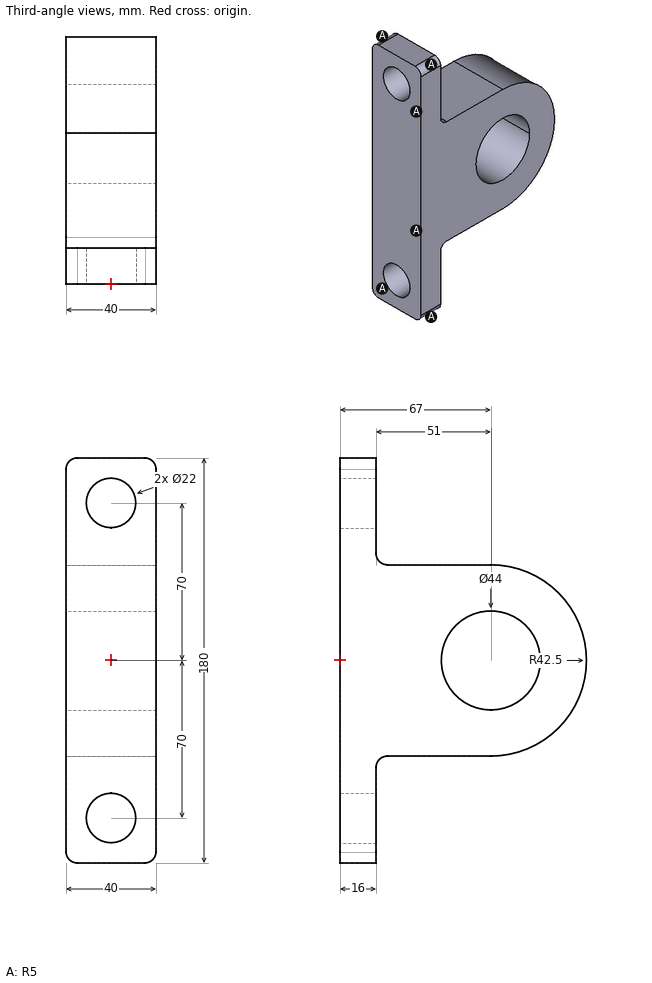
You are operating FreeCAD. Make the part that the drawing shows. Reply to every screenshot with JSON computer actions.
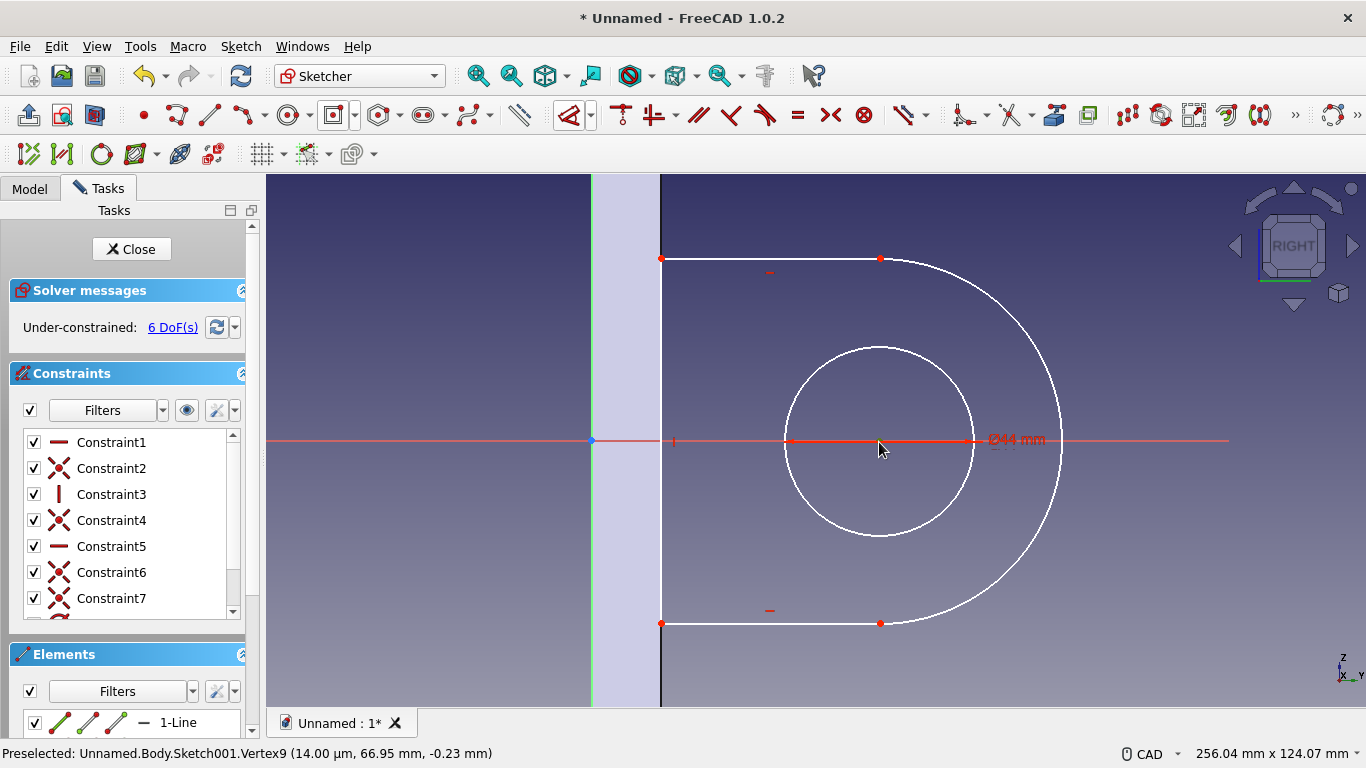
{"action": "left_click", "coordinate": [359, 440]}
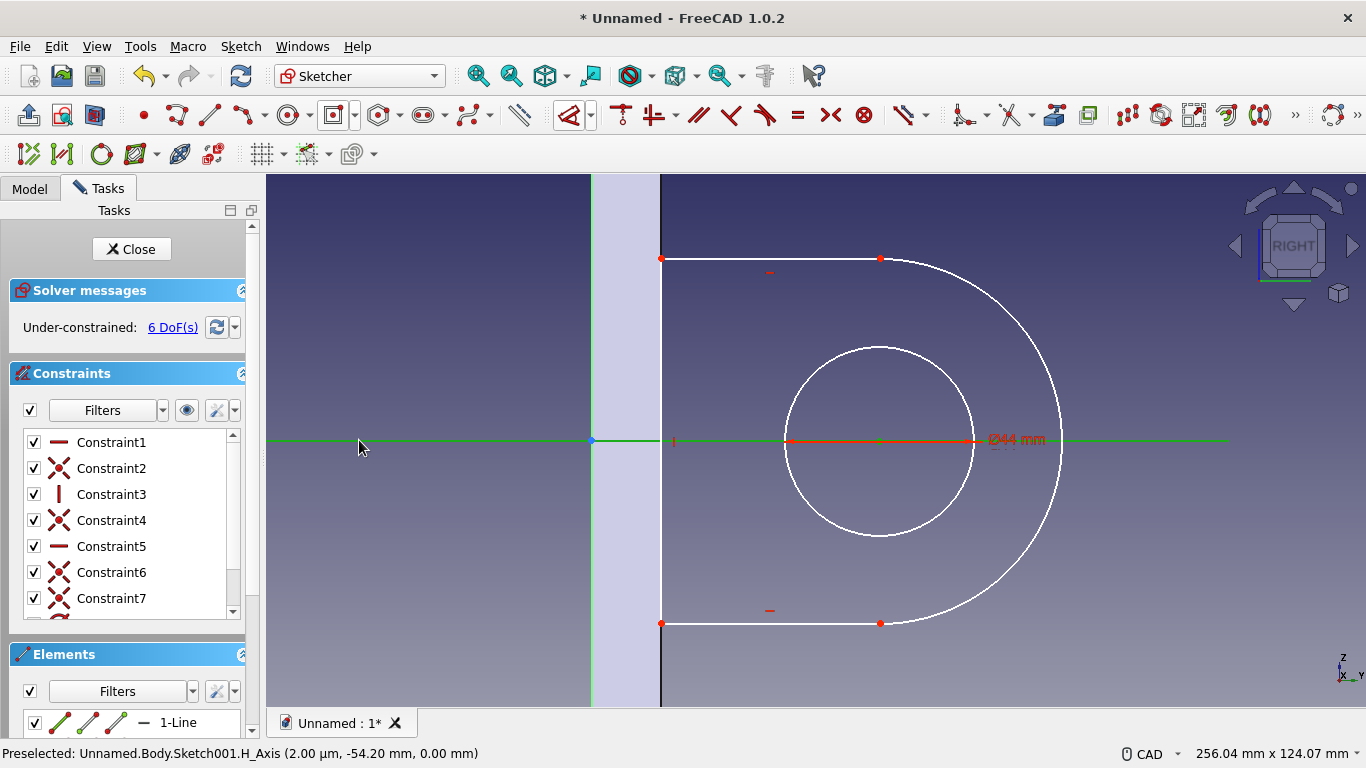
{"action": "key", "text": "c"}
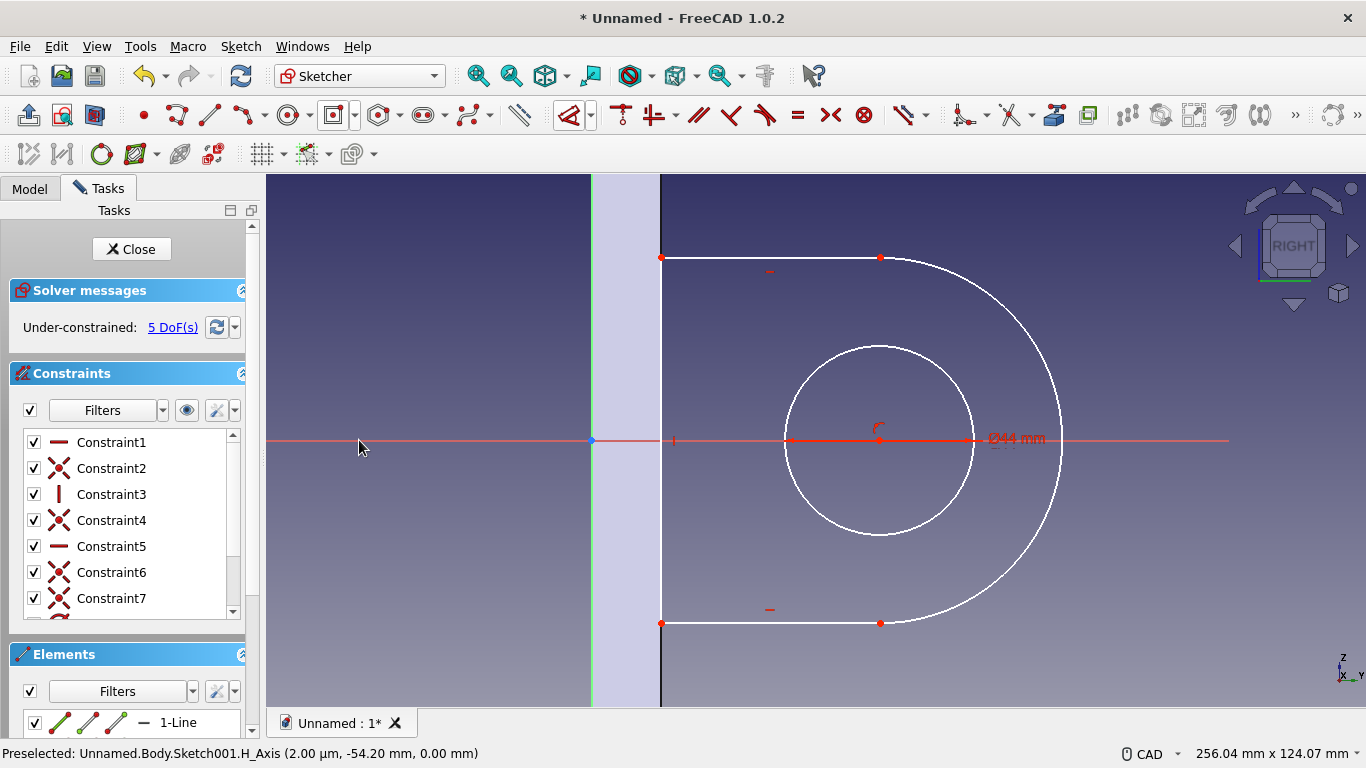
{"action": "left_click", "coordinate": [1027, 548]}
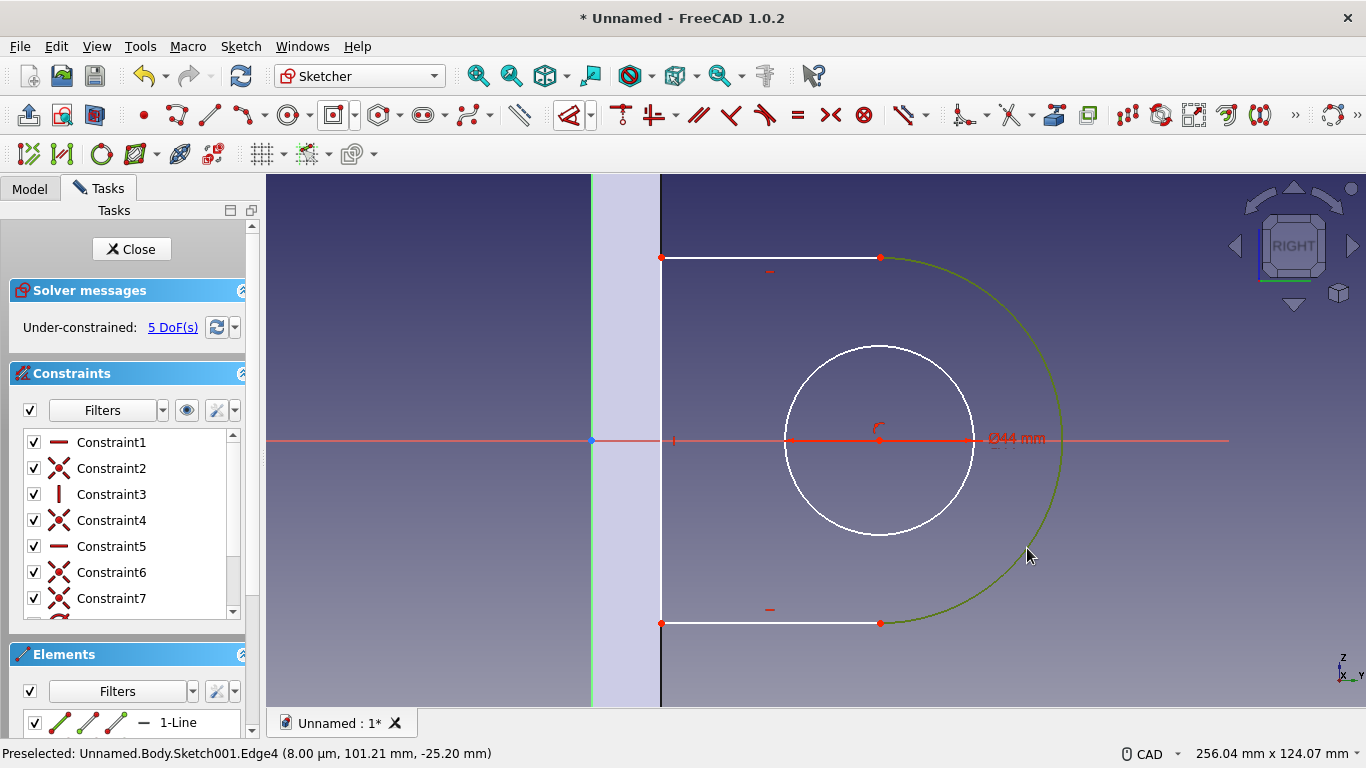
{"action": "key", "text": "k r"}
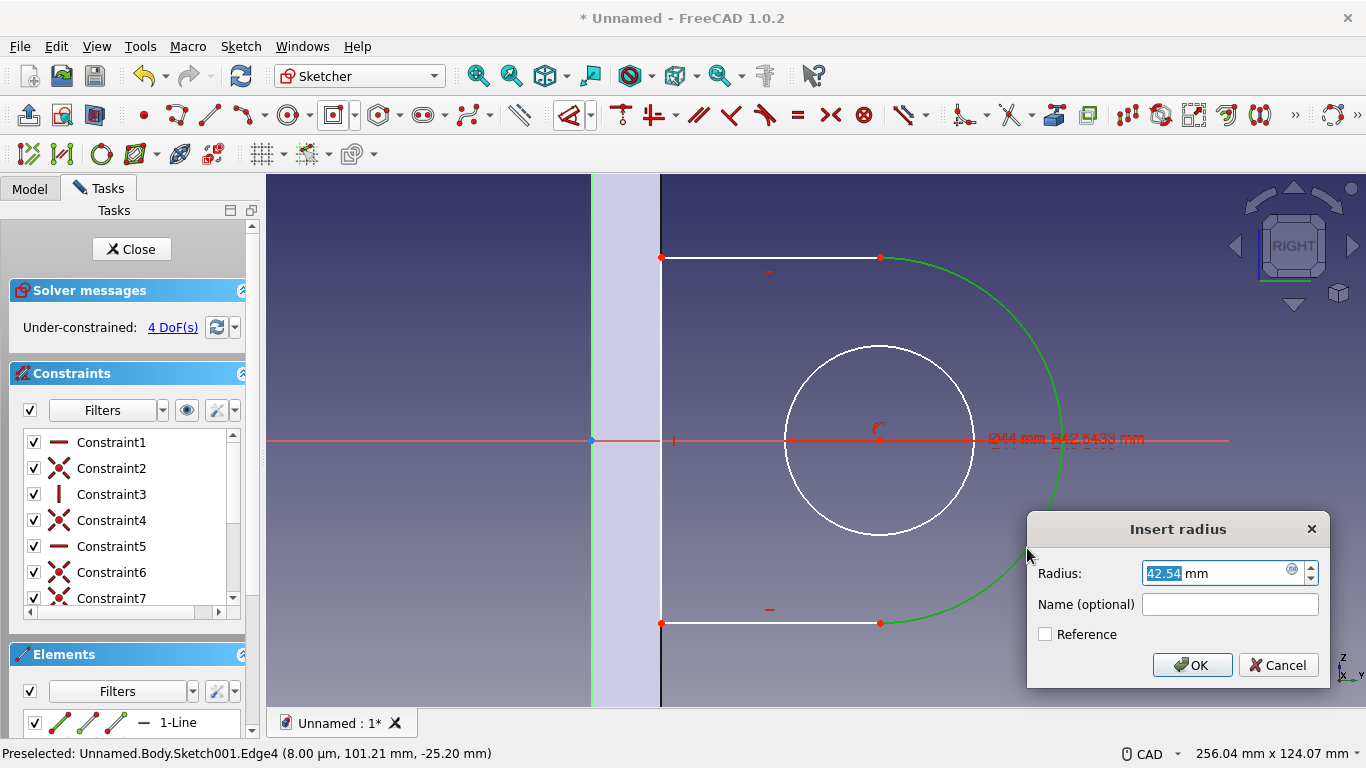
{"action": "type", "text": "42.5"}
{"action": "key", "text": "Return"}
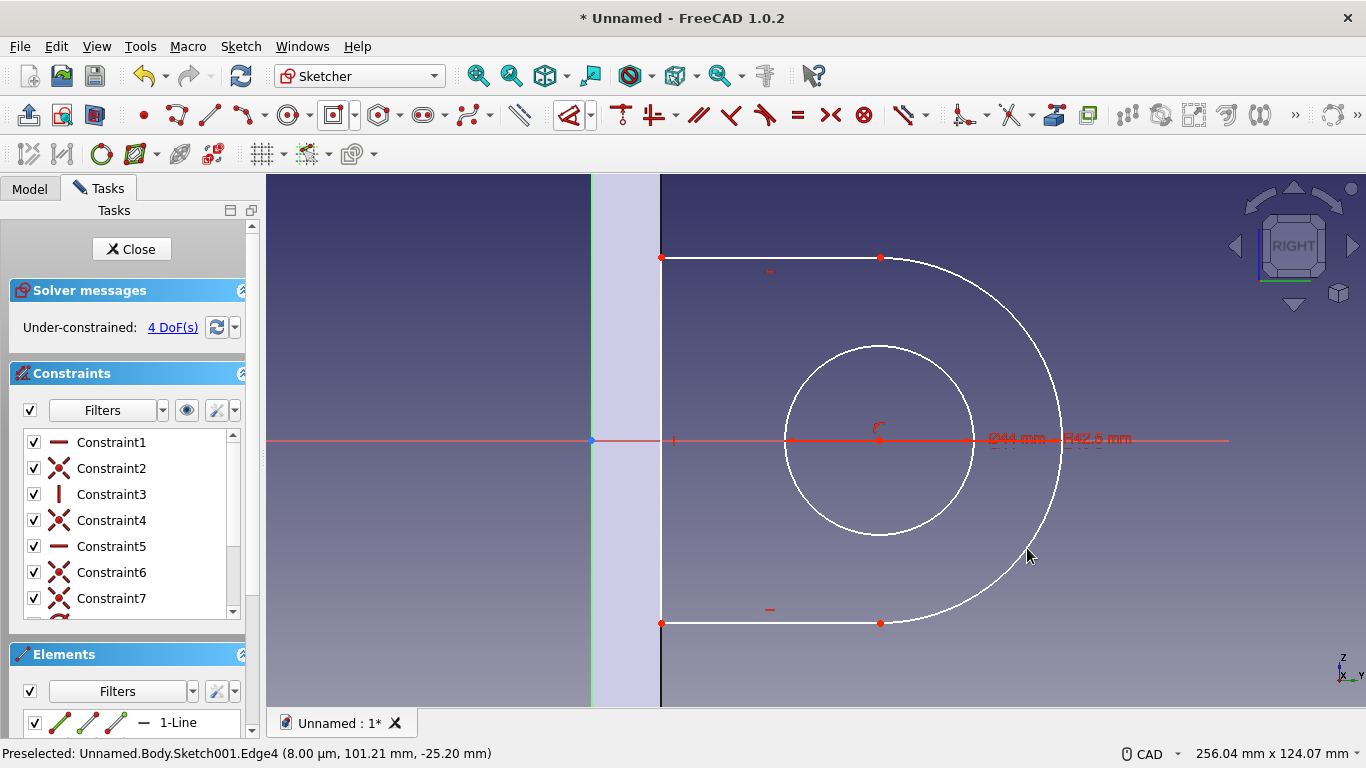
{"action": "left_click", "coordinate": [814, 258]}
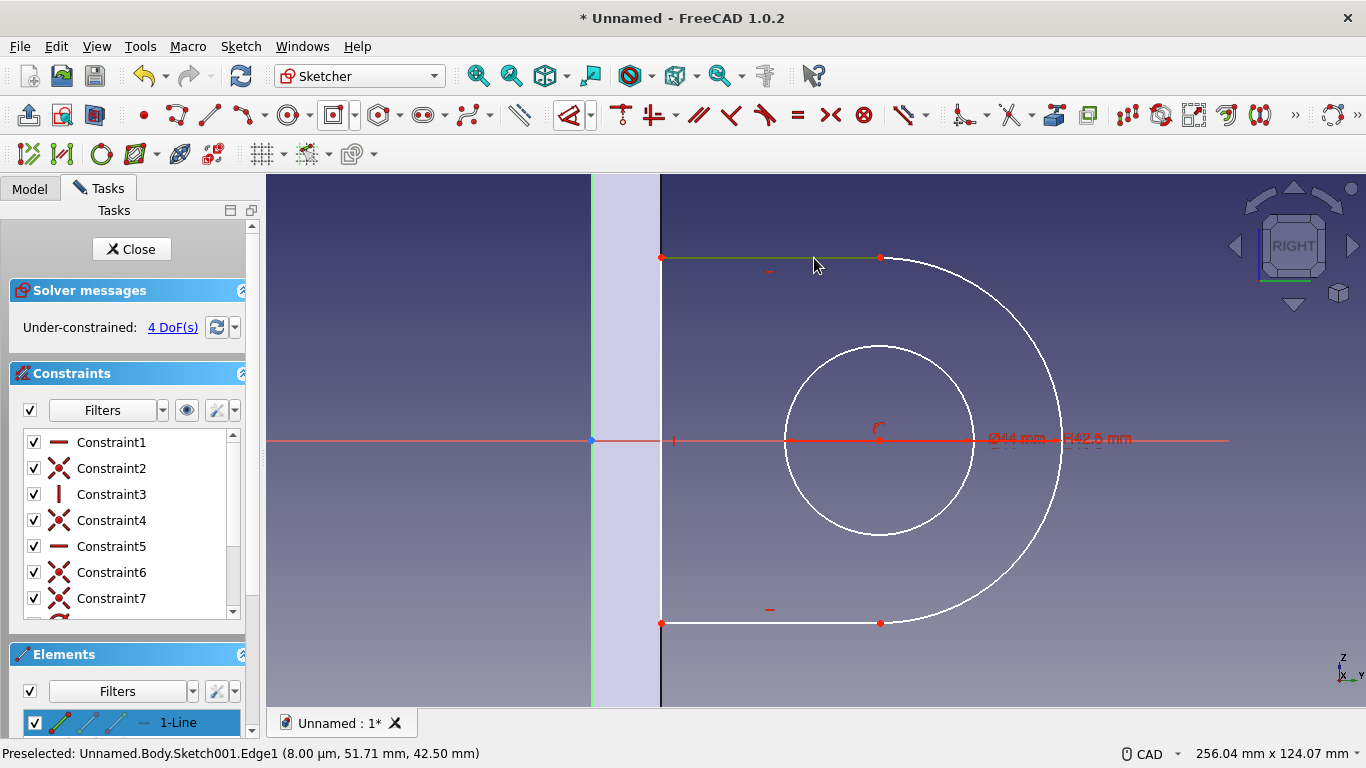
{"action": "key", "text": "l"}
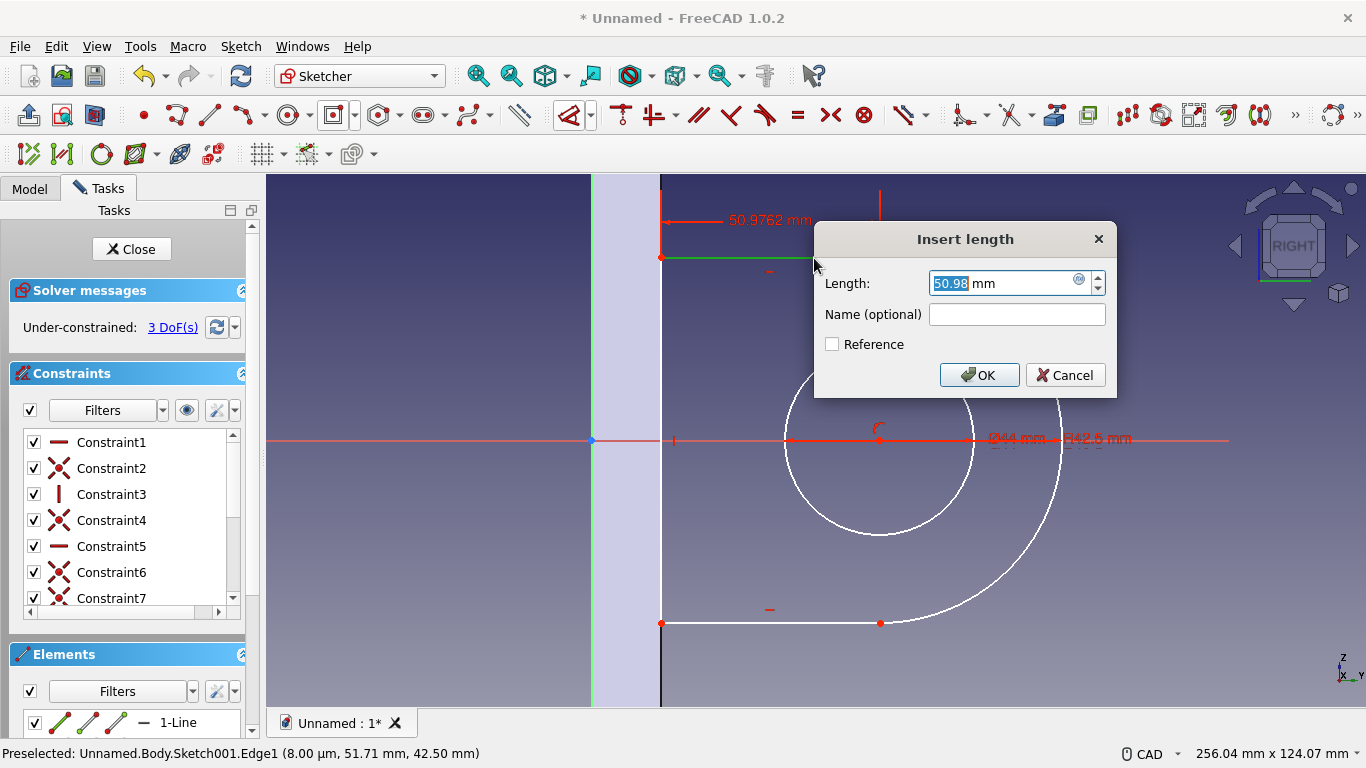
{"action": "type", "text": "51"}
{"action": "key", "text": "Return"}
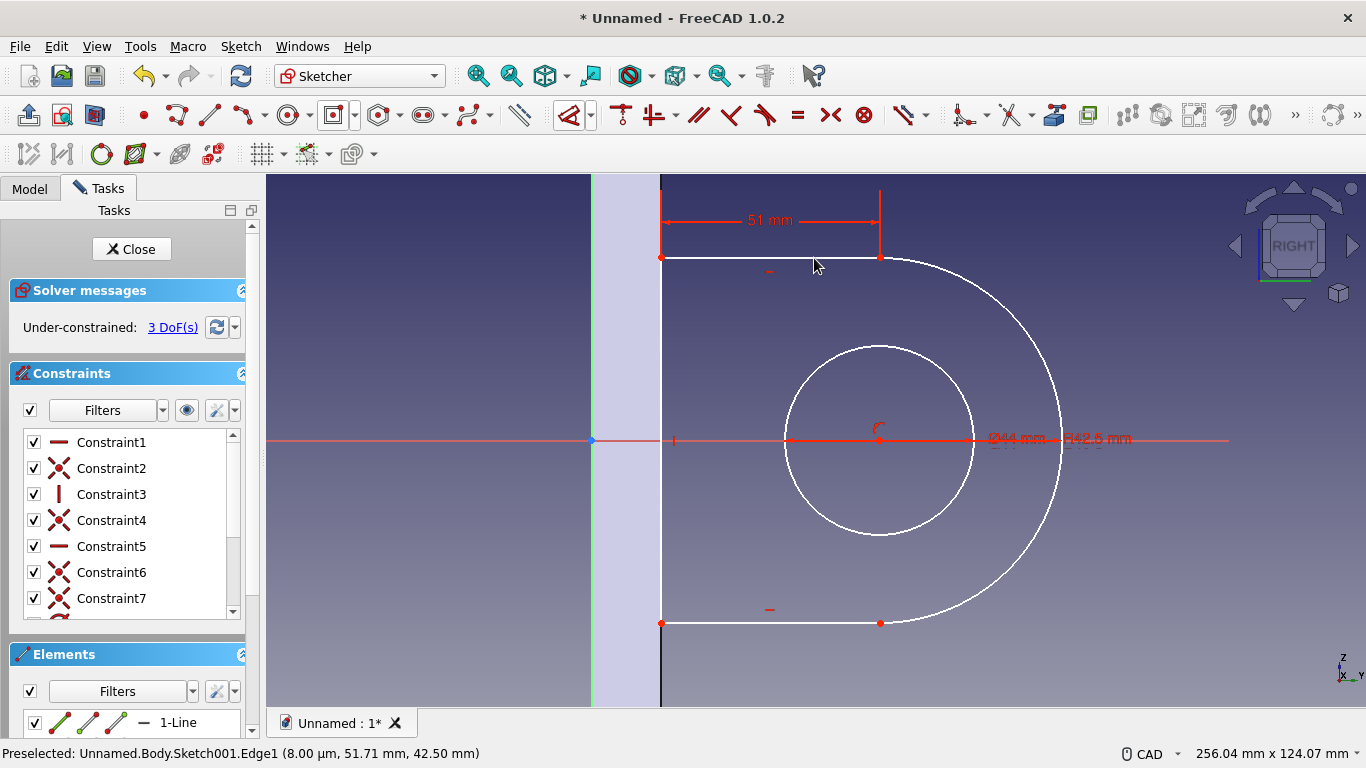
{"action": "left_click", "coordinate": [727, 623]}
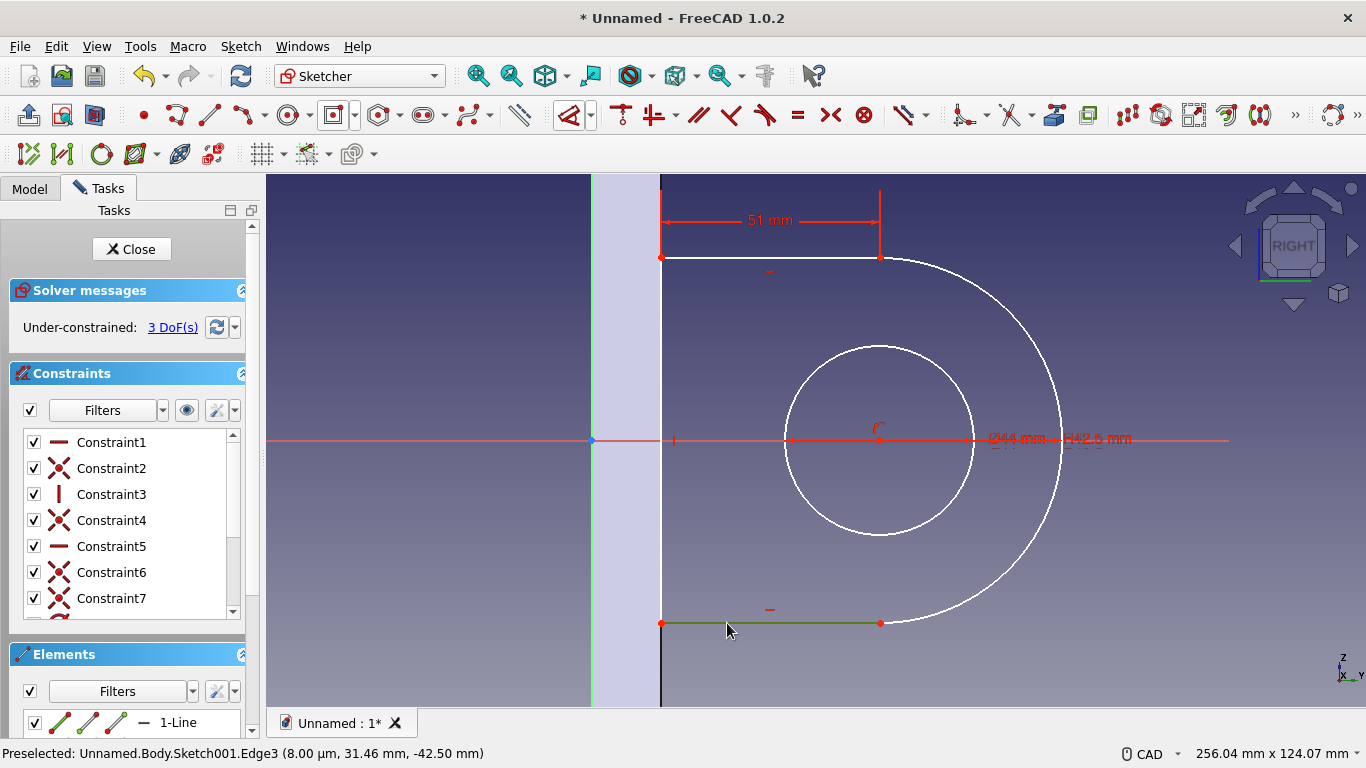
{"action": "key", "text": "l"}